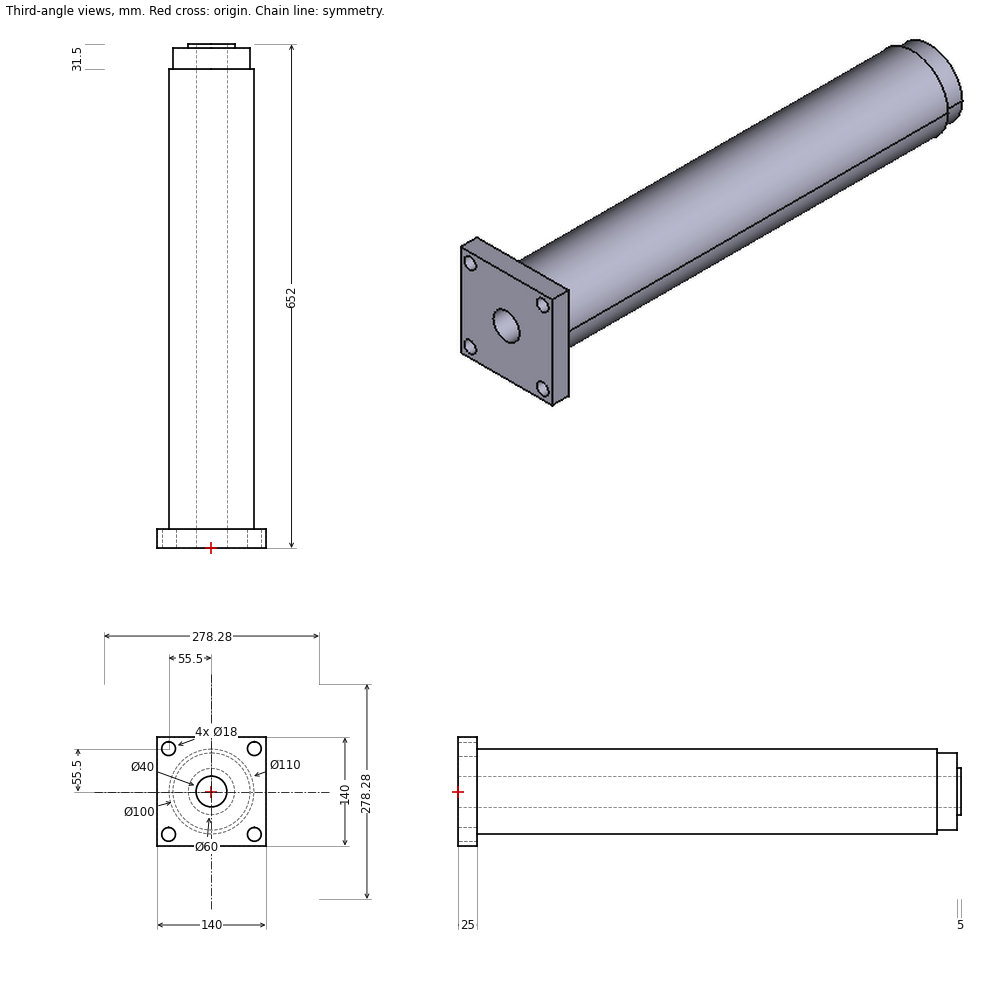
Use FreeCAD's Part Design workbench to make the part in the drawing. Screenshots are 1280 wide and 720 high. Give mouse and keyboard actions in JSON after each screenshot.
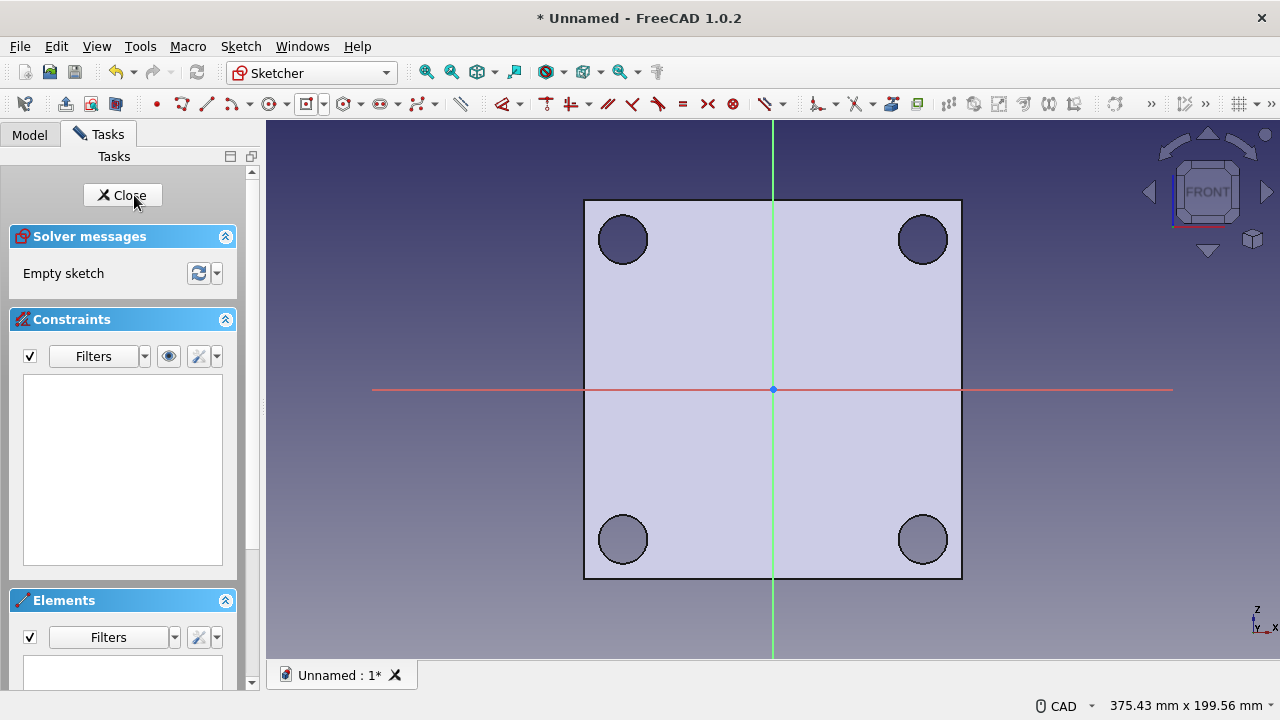
{"action": "left_click", "coordinate": [268, 104]}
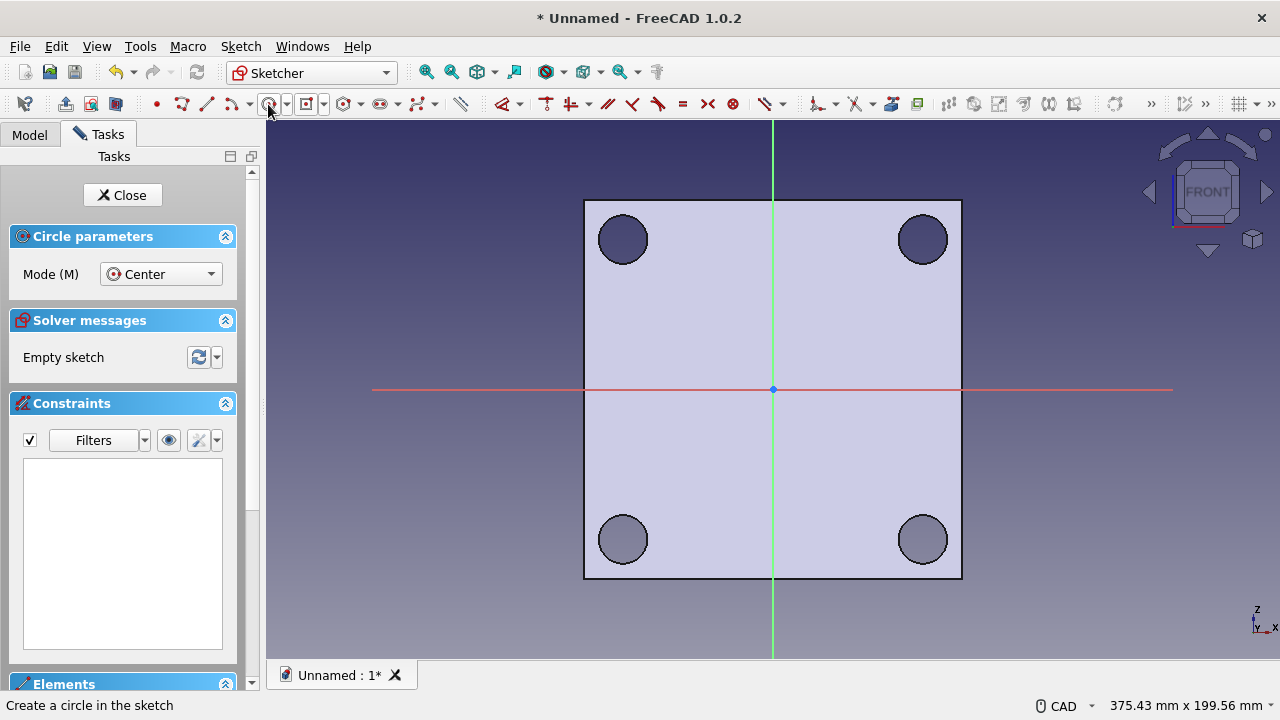
{"action": "left_click", "coordinate": [773, 390]}
{"action": "mouse_move", "coordinate": [878, 284]}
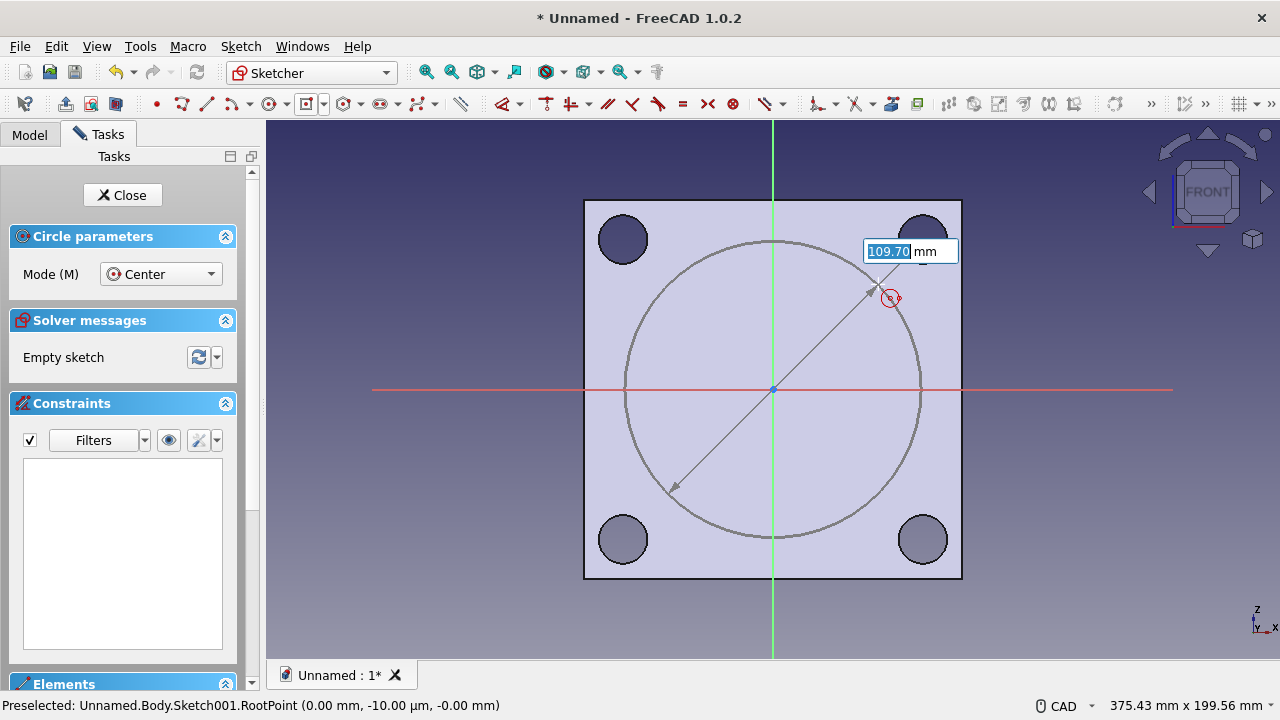
{"action": "type", "text": "110"}
{"action": "key", "text": "Return"}
{"action": "key", "text": "Escape"}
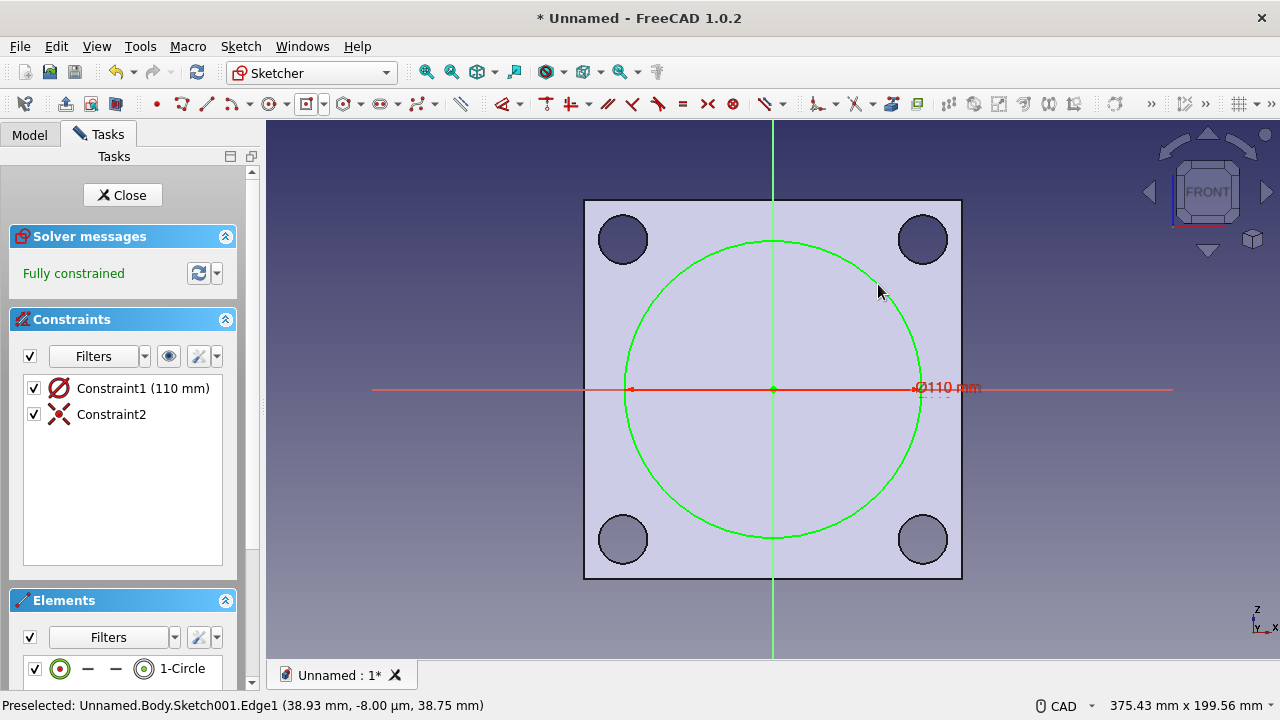
{"action": "left_click", "coordinate": [123, 195]}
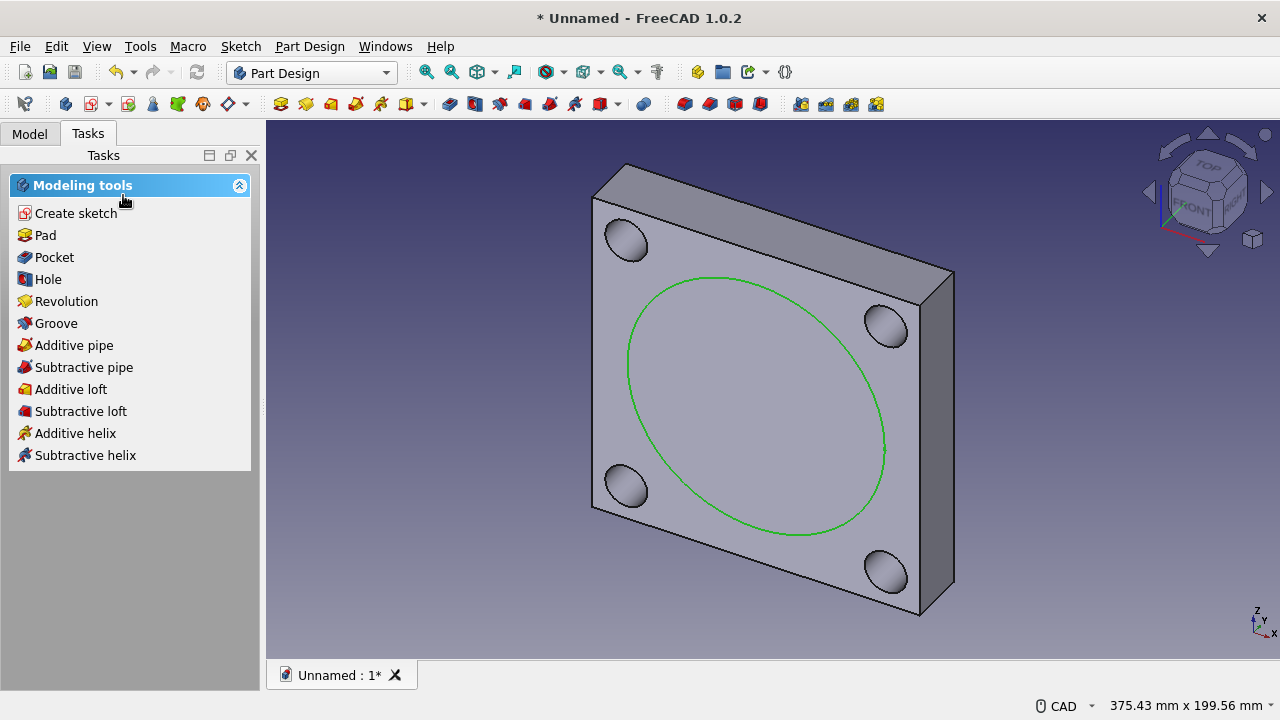
{"action": "left_click", "coordinate": [281, 104]}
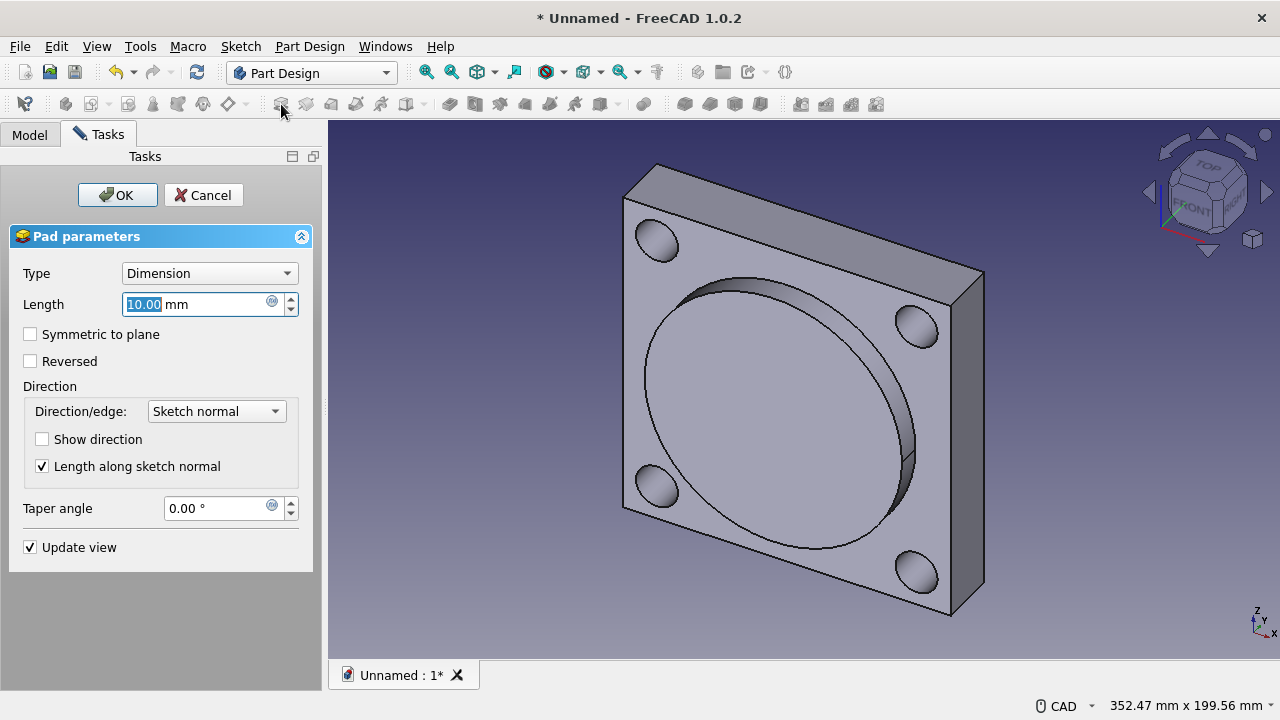
{"action": "type", "text": "652"}
{"action": "key", "text": "Tab"}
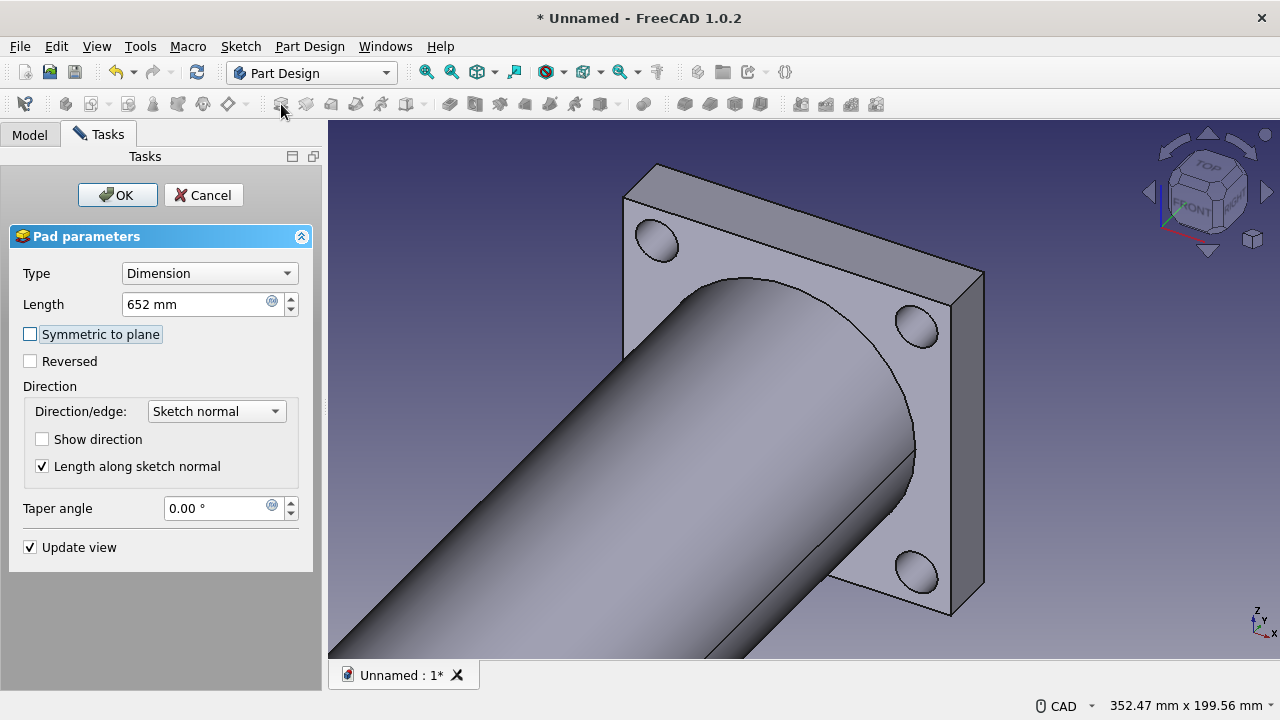
{"action": "left_click", "coordinate": [31, 361]}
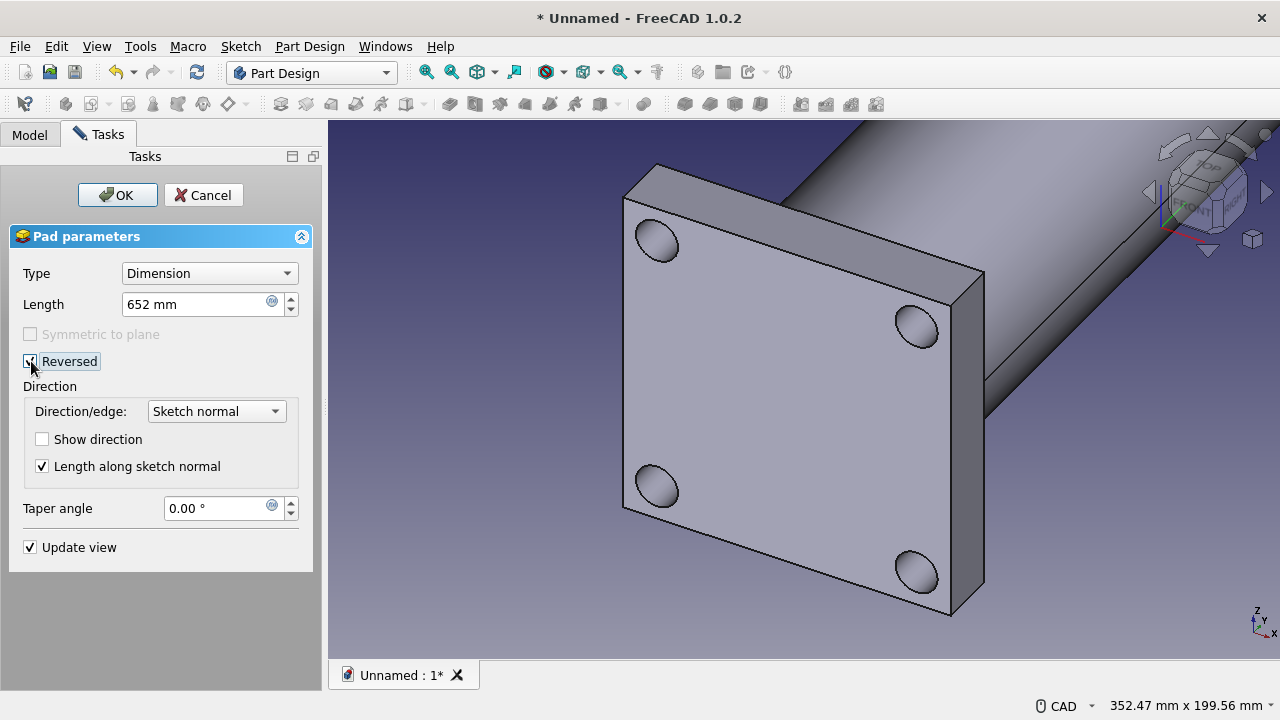
{"action": "left_click", "coordinate": [118, 195]}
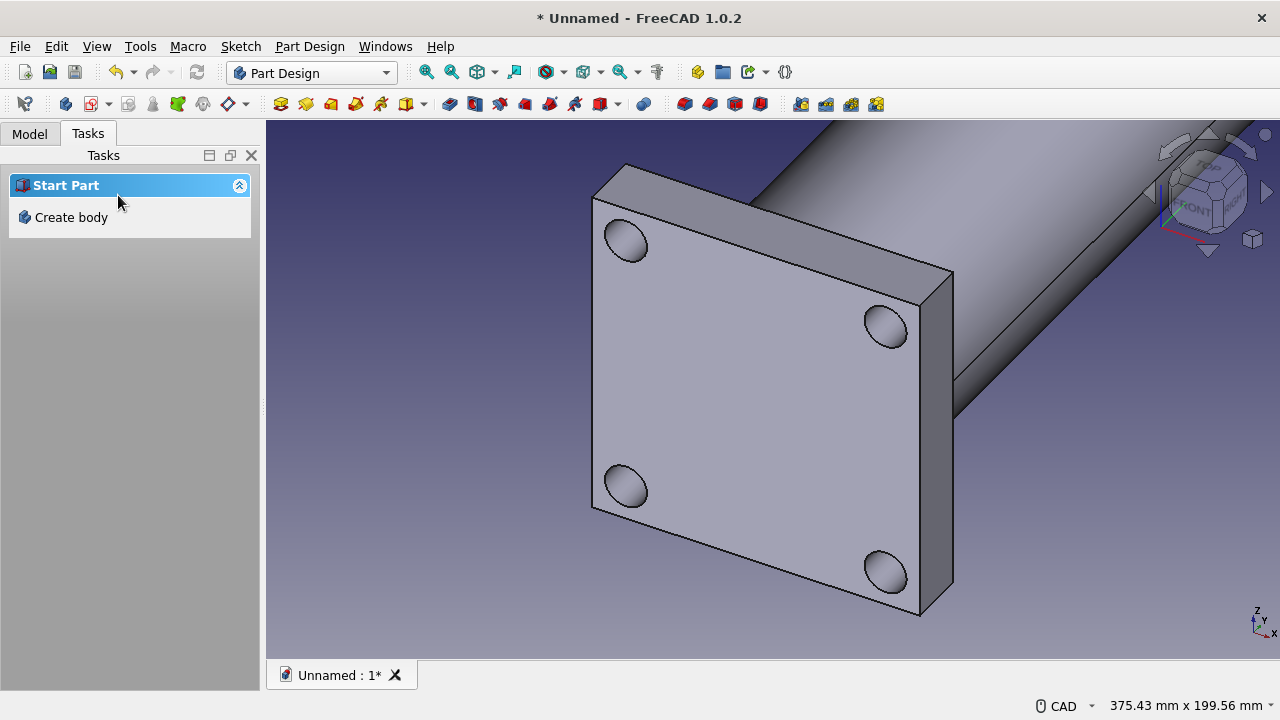
{"action": "left_click", "coordinate": [427, 72]}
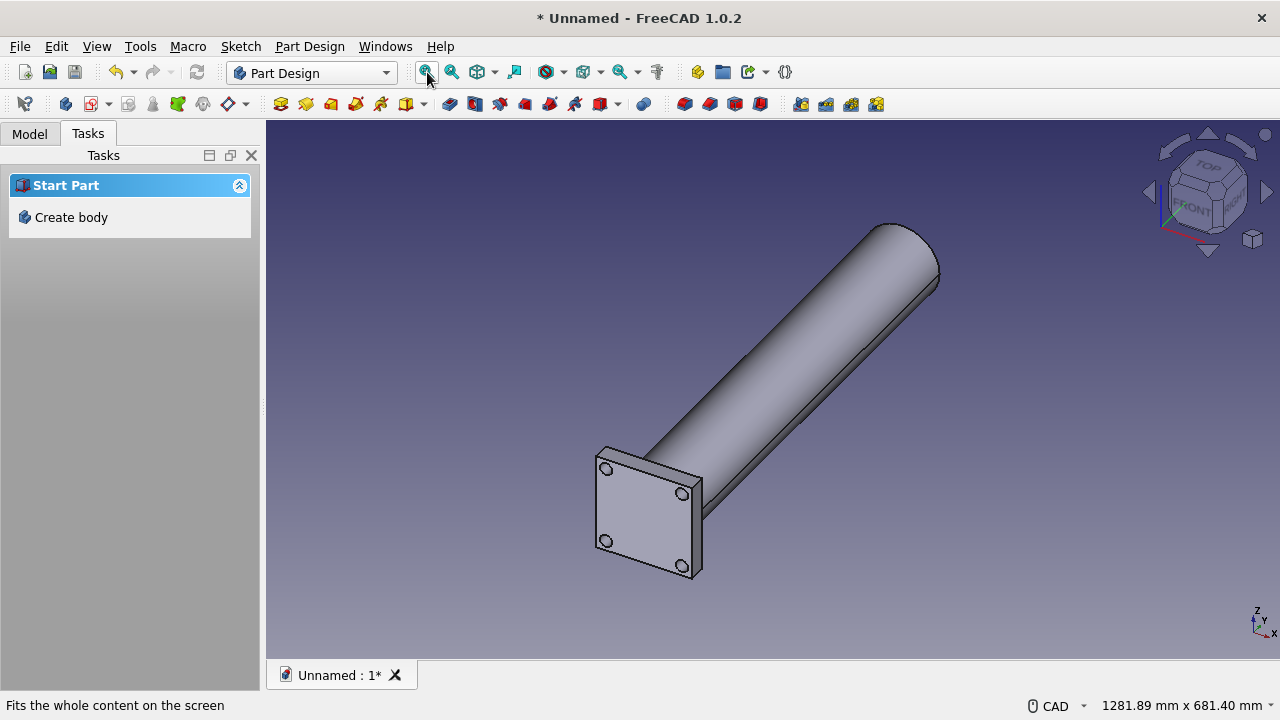
{"action": "key", "text": "4"}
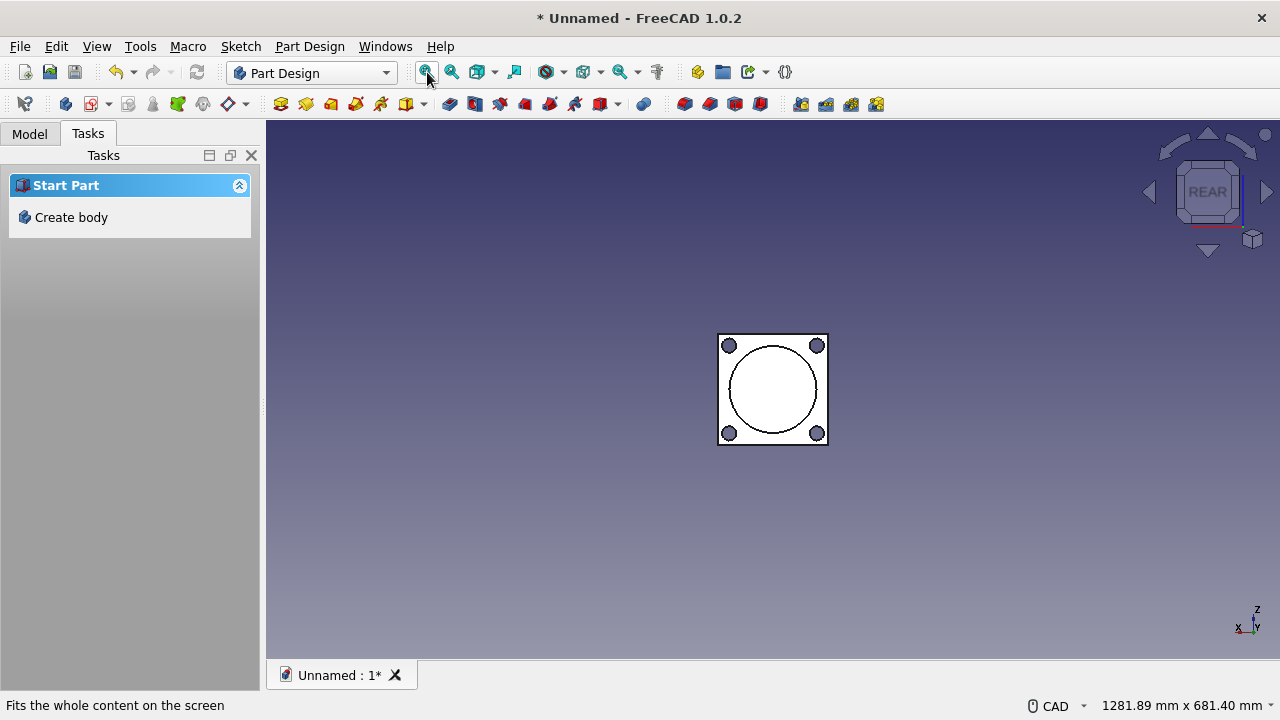
{"action": "left_click", "coordinate": [427, 72]}